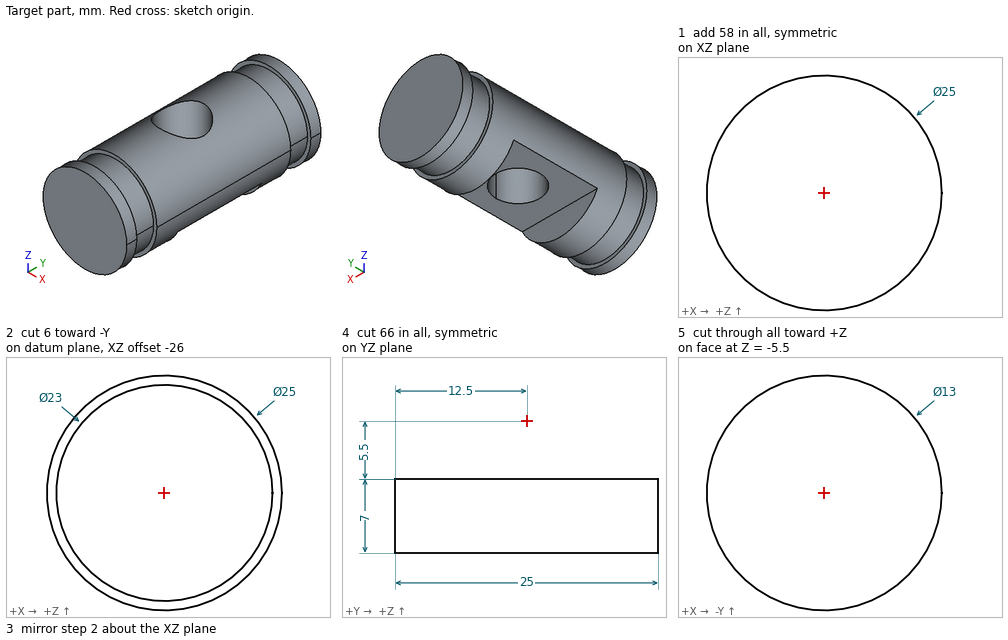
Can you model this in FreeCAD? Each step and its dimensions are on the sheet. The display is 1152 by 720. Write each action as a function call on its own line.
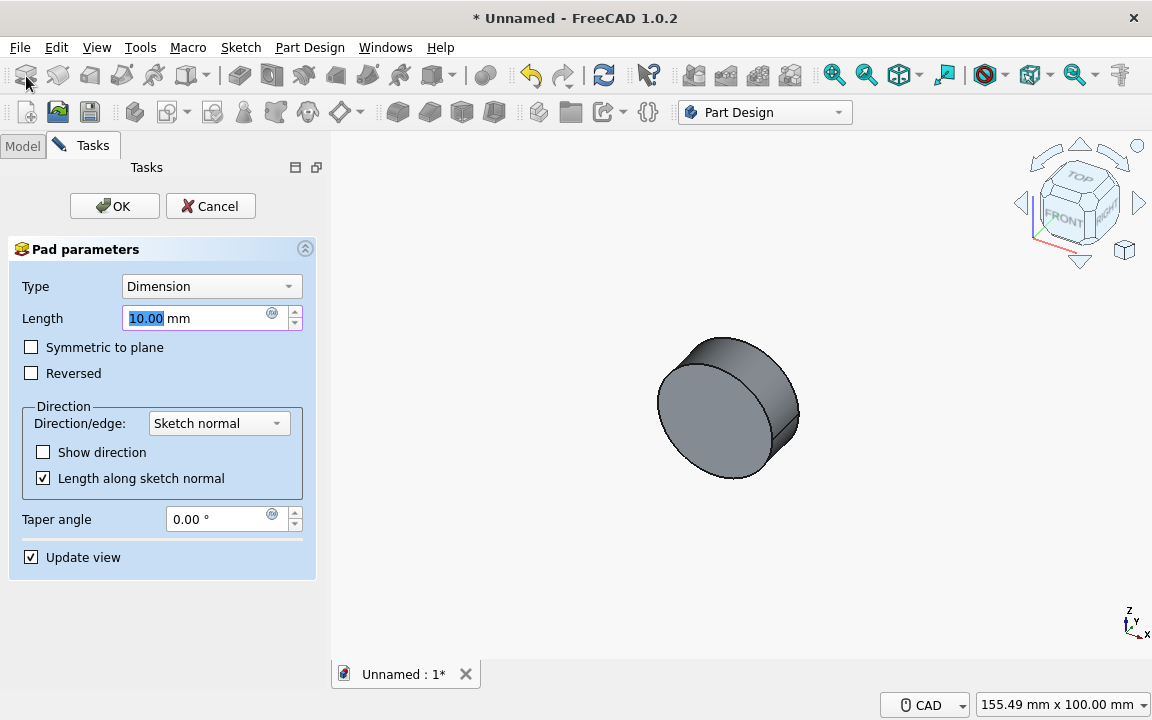
text(58)
key(Tab)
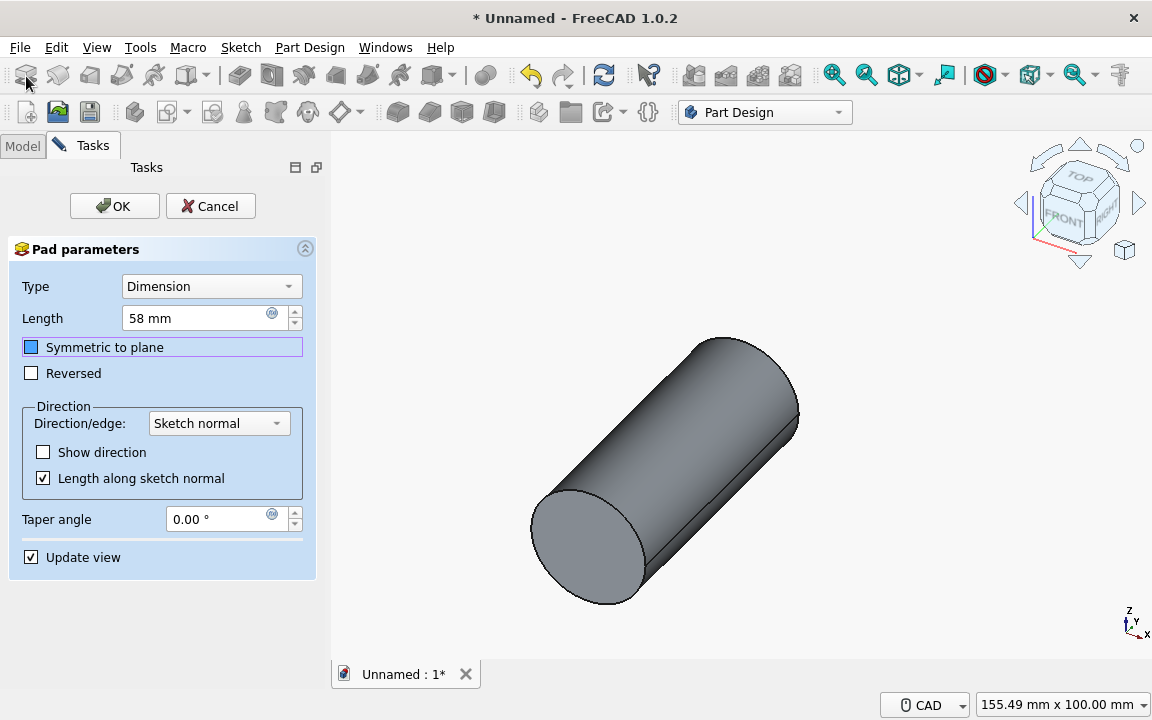
click(30, 347)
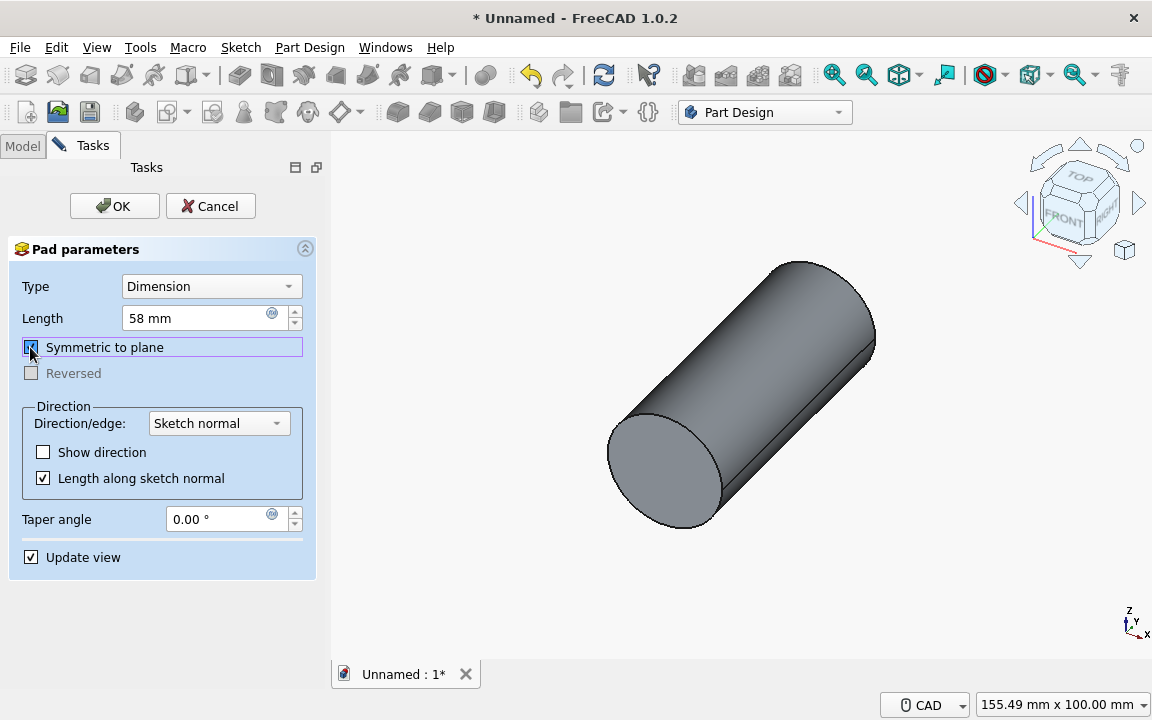
click(115, 206)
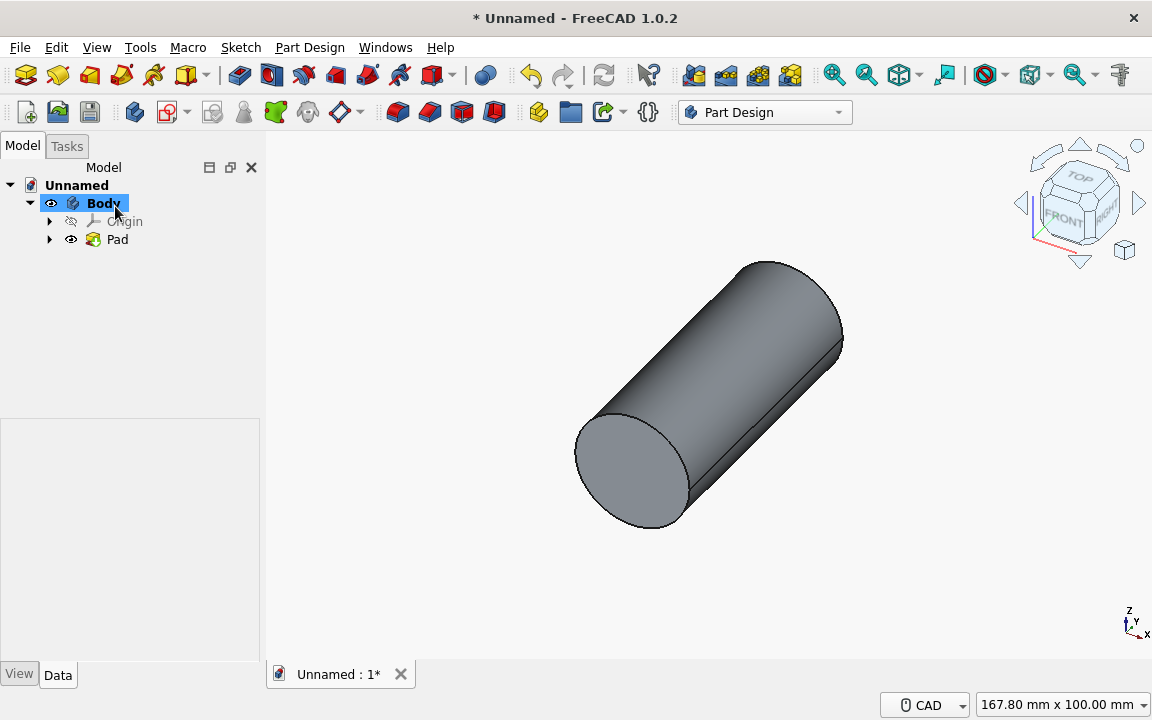
click(50, 221)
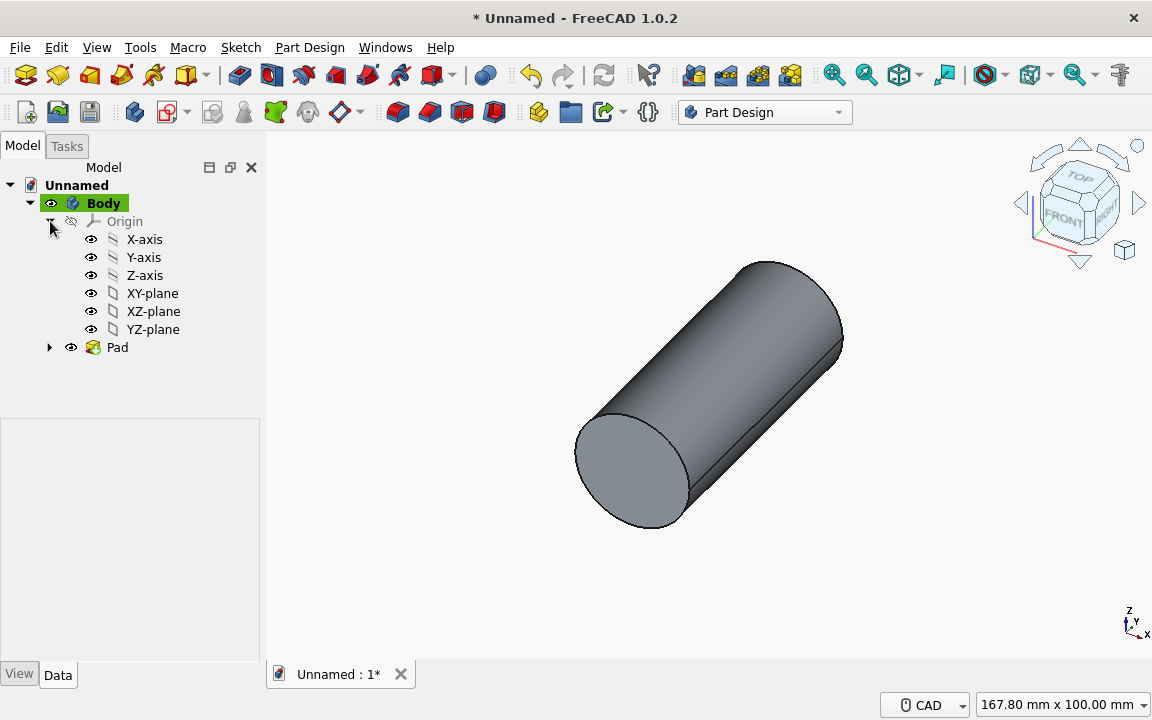
click(136, 311)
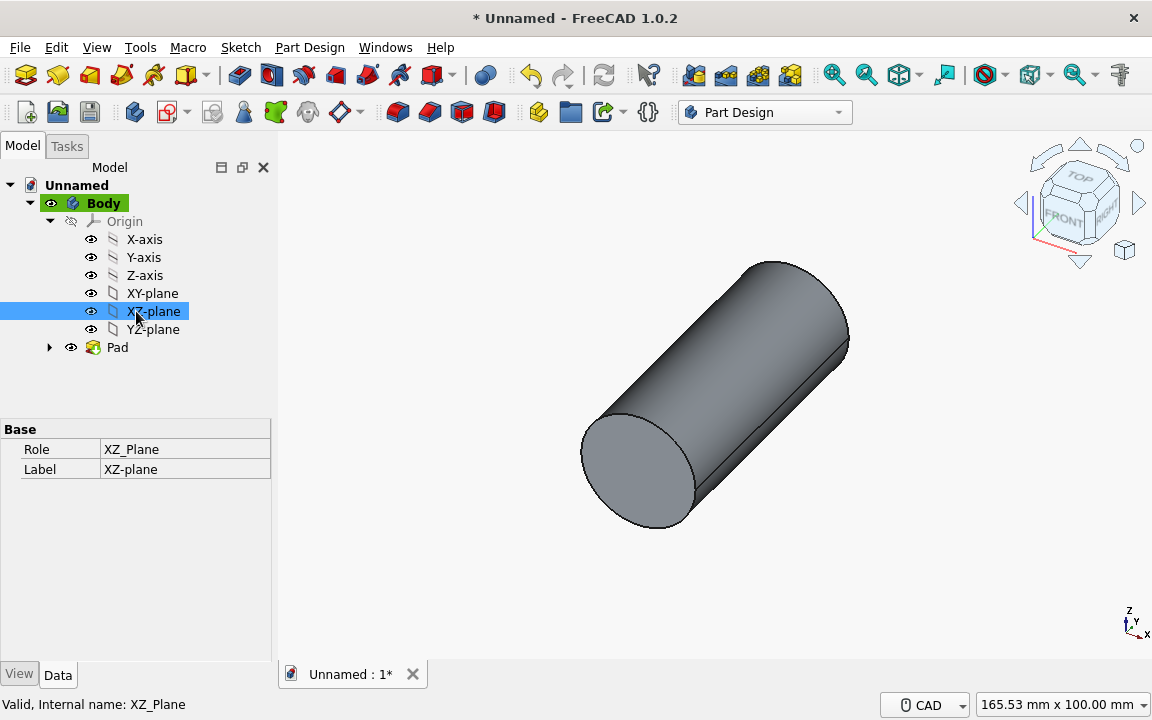
click(340, 112)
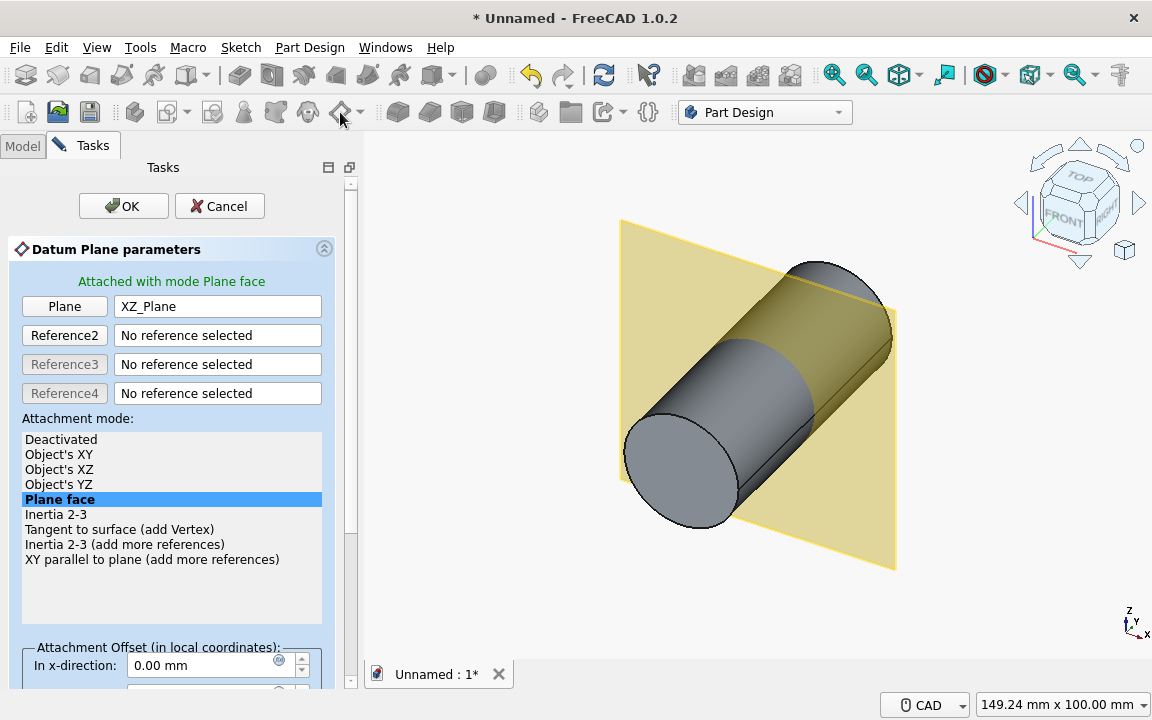
scroll(351, 432, down, 2)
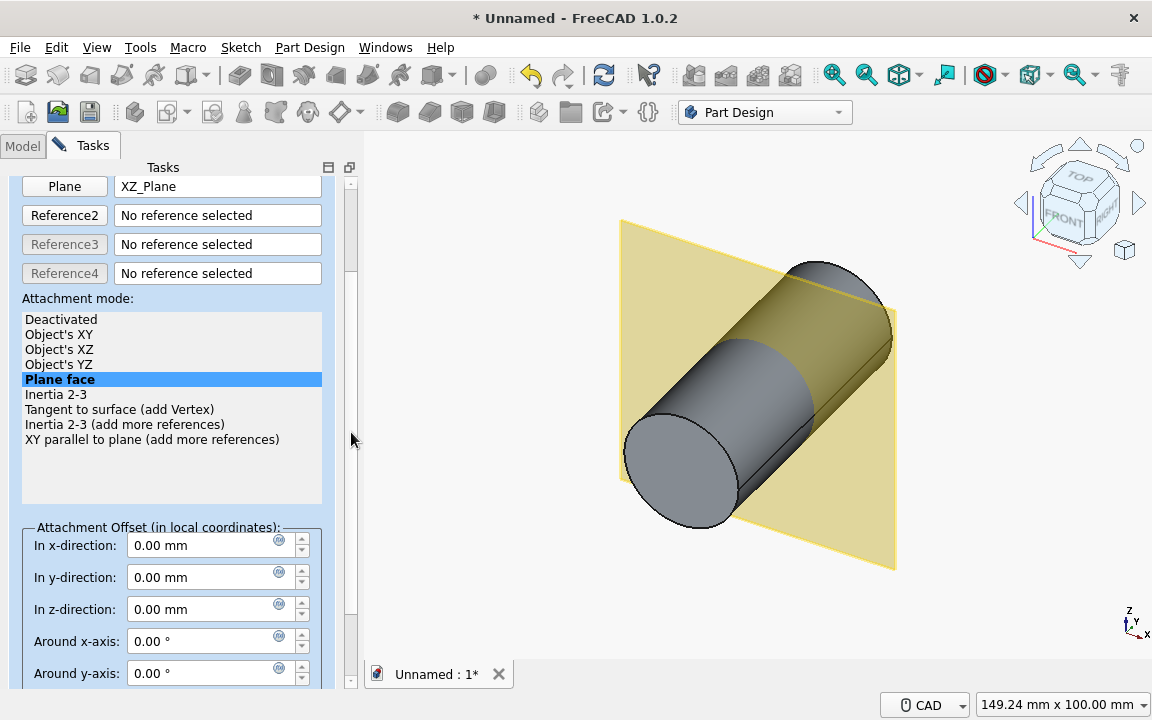
triple_click(210, 609)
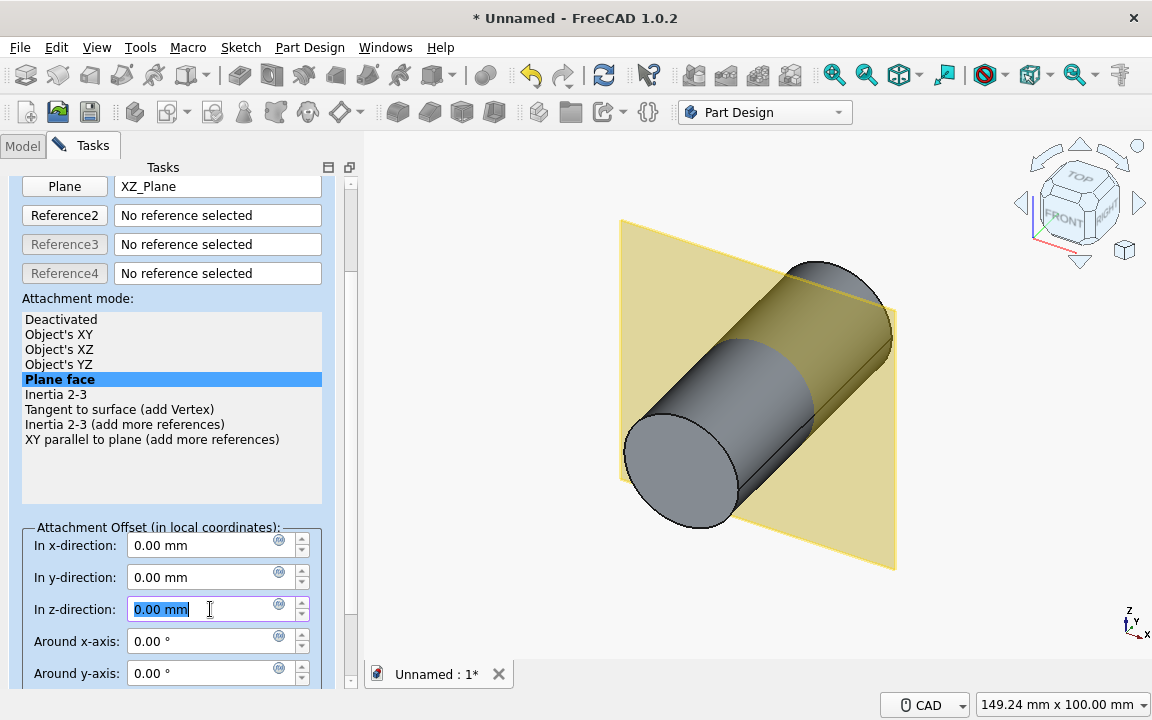
text(-26)
key(Tab)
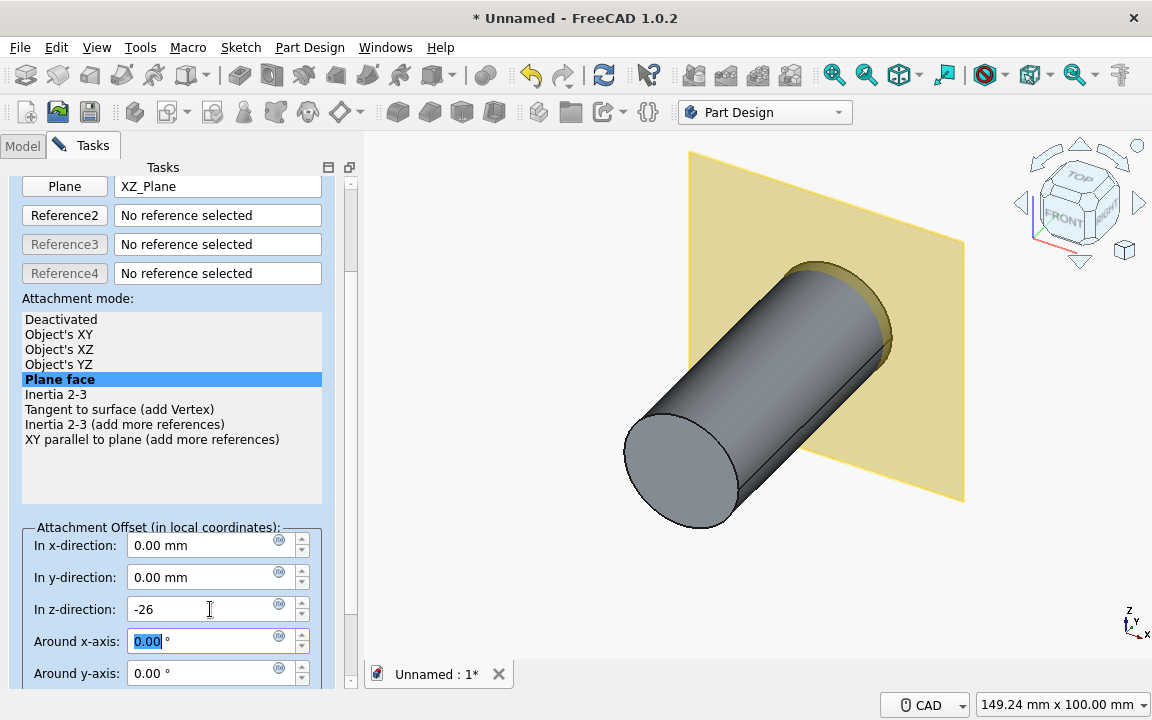
scroll(351, 432, up, 3)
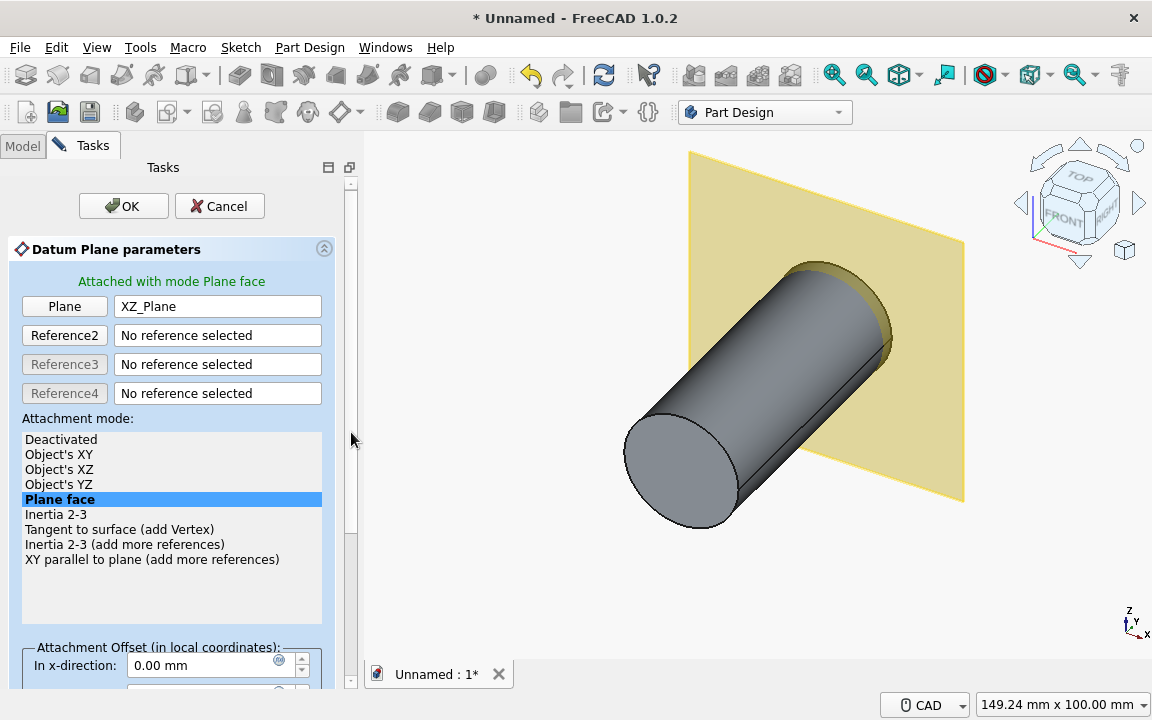
click(124, 206)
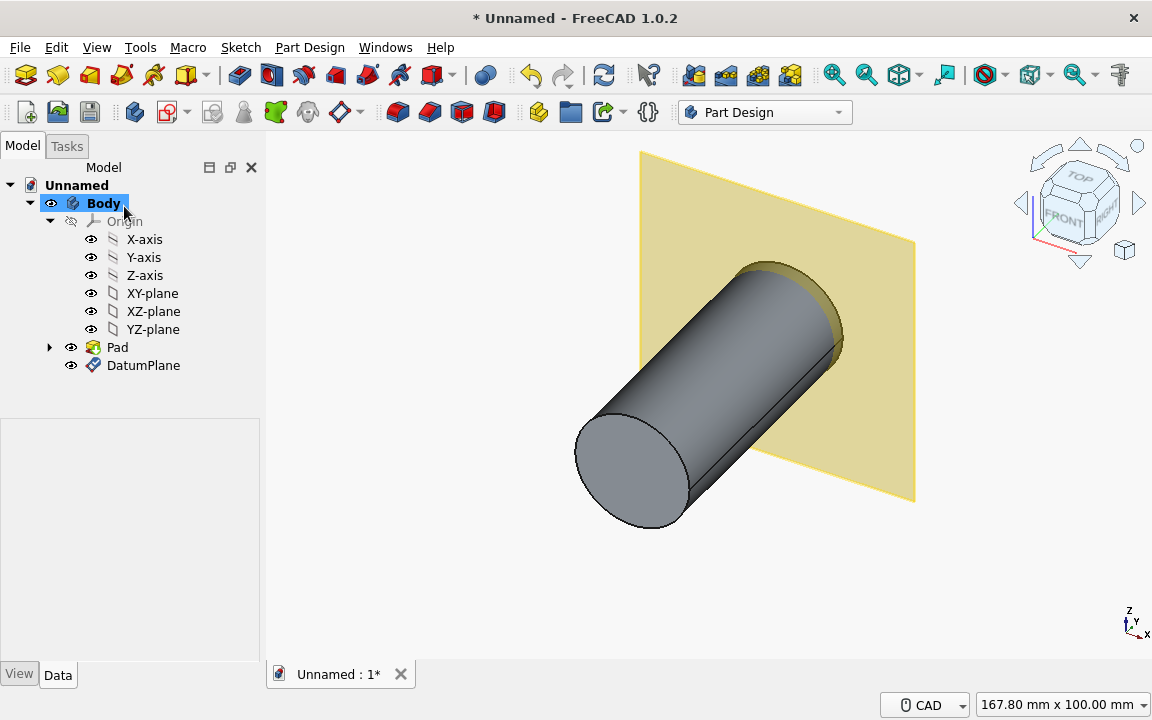
click(116, 365)